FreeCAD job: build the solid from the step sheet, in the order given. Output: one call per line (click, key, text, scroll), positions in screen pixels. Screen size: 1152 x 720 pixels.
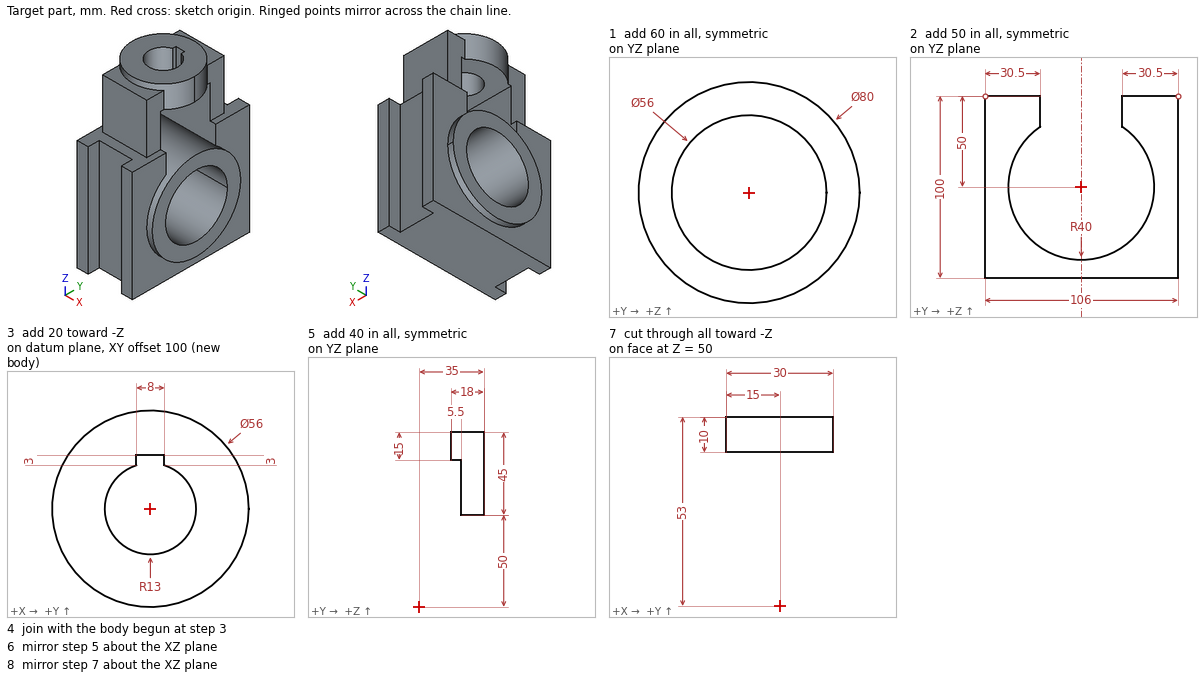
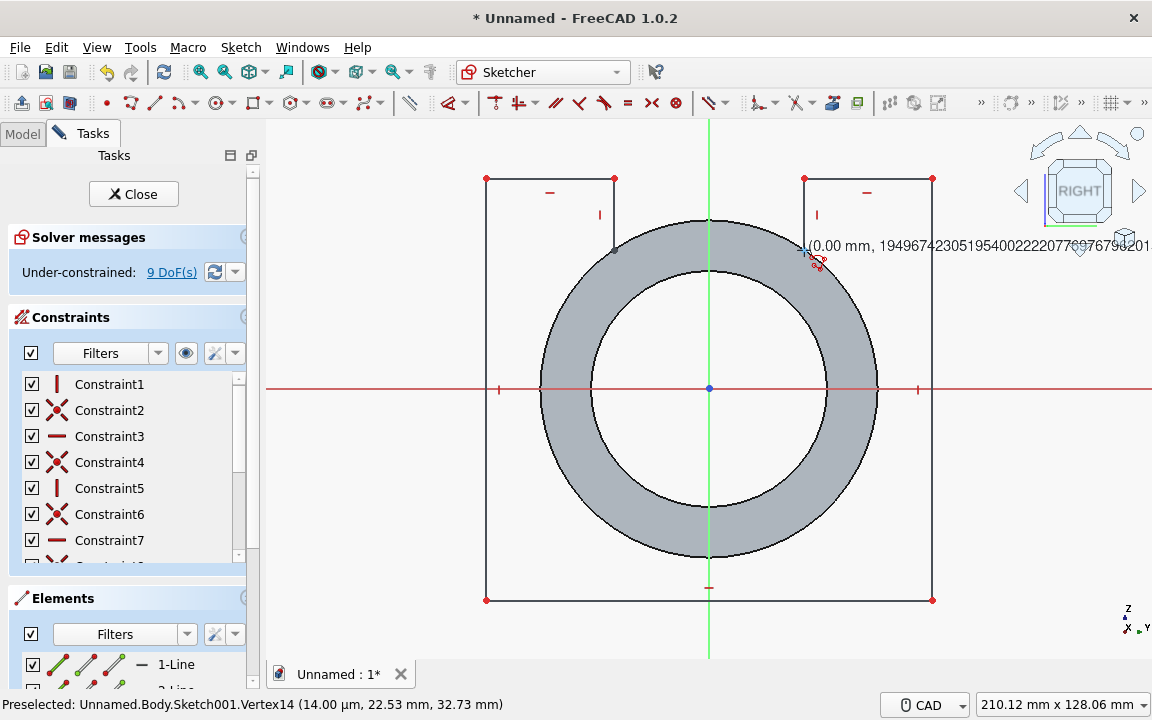
click(198, 104)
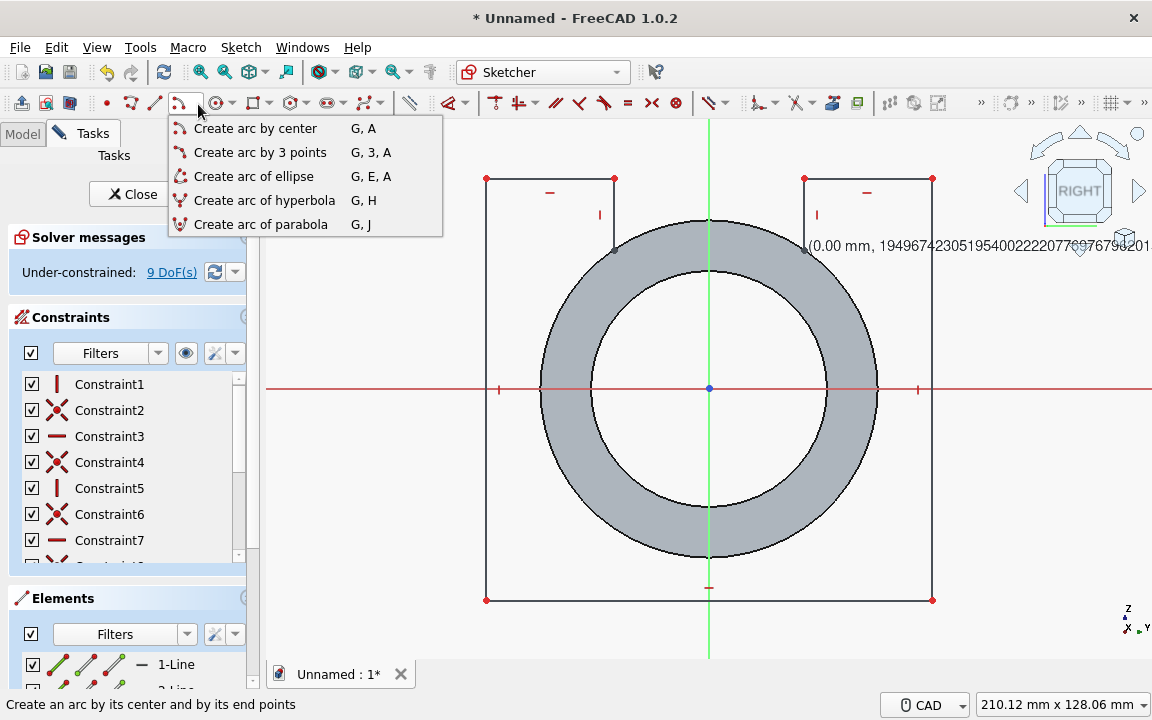
click(306, 152)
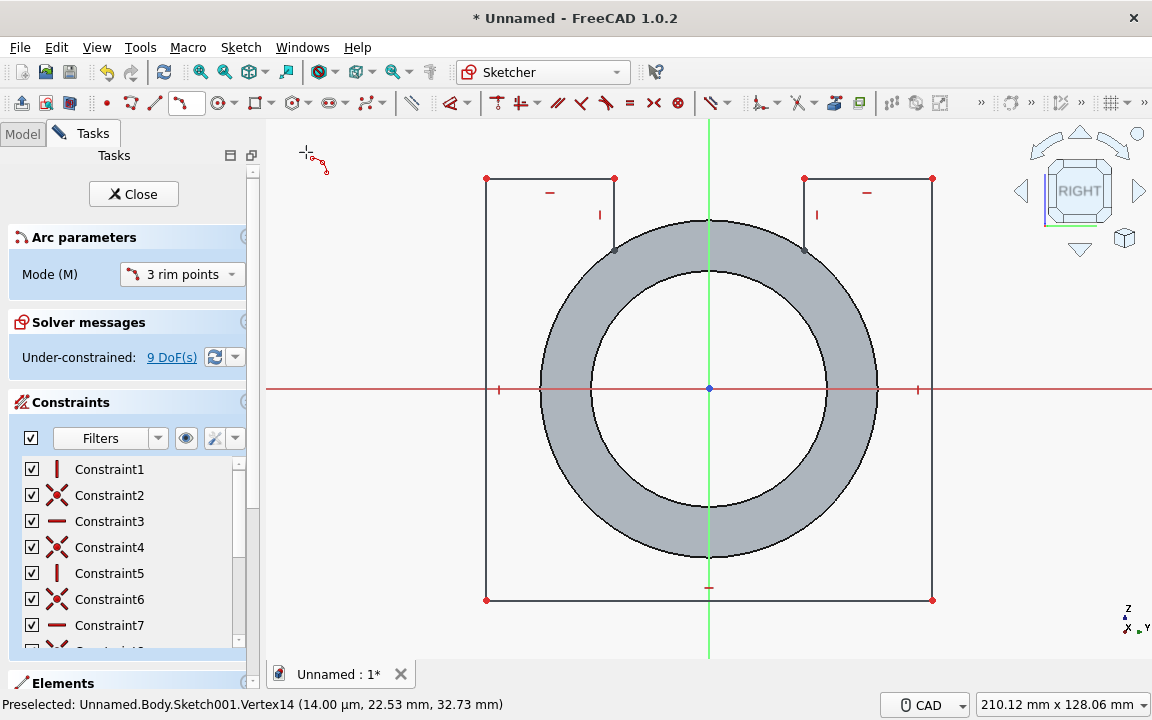
click(804, 251)
click(614, 251)
click(627, 536)
key(Escape)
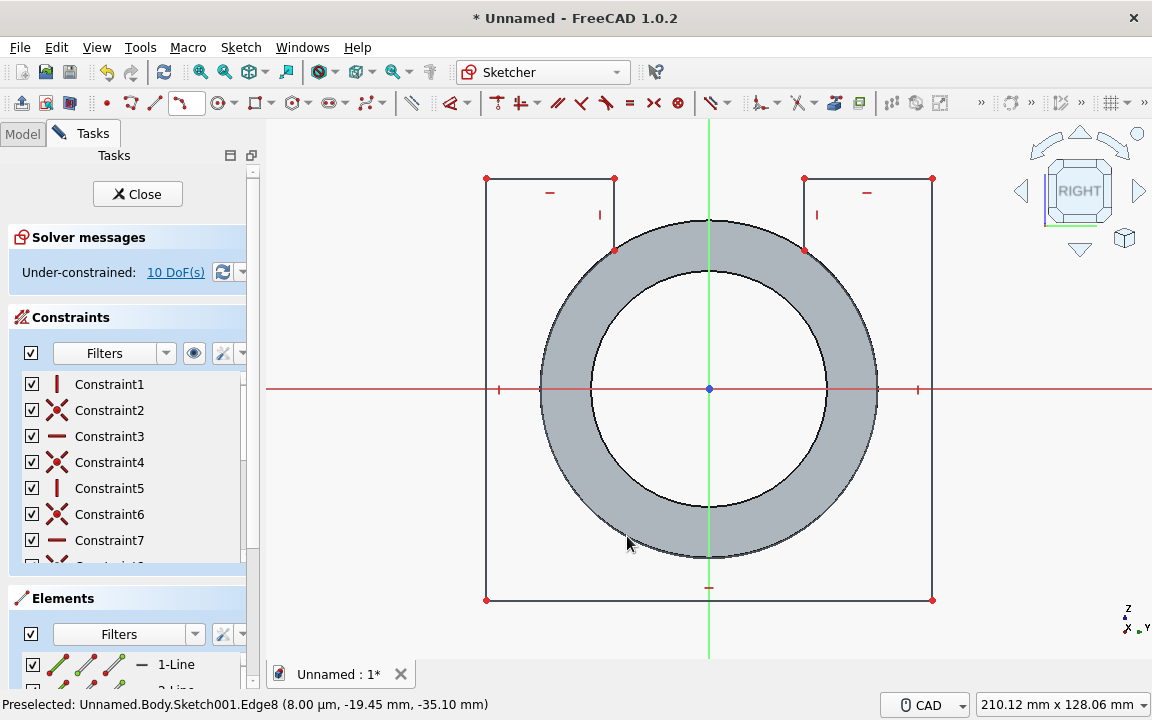
drag(699, 379, 719, 400)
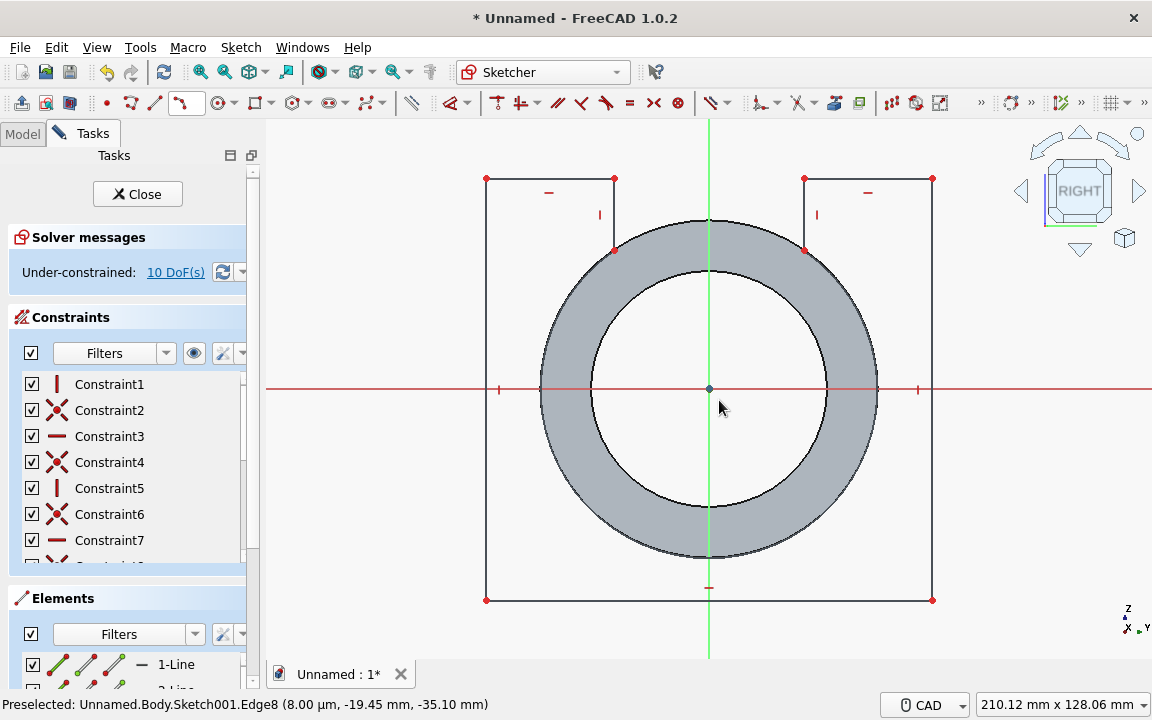
click(498, 104)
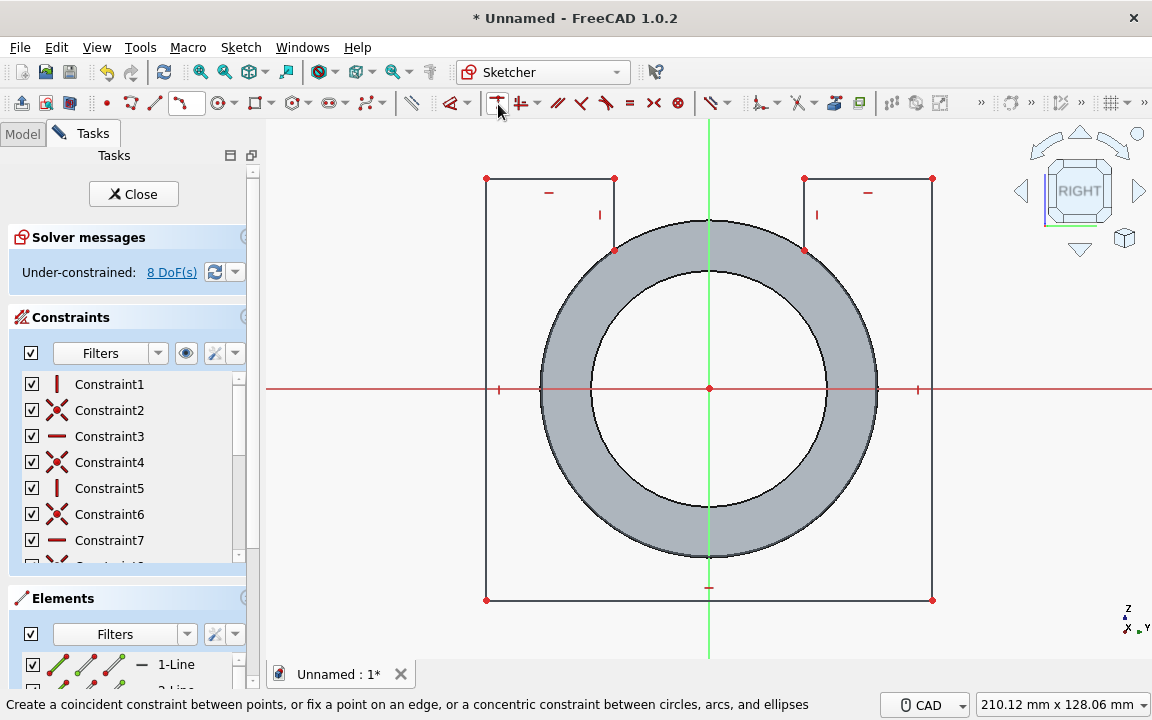
click(486, 179)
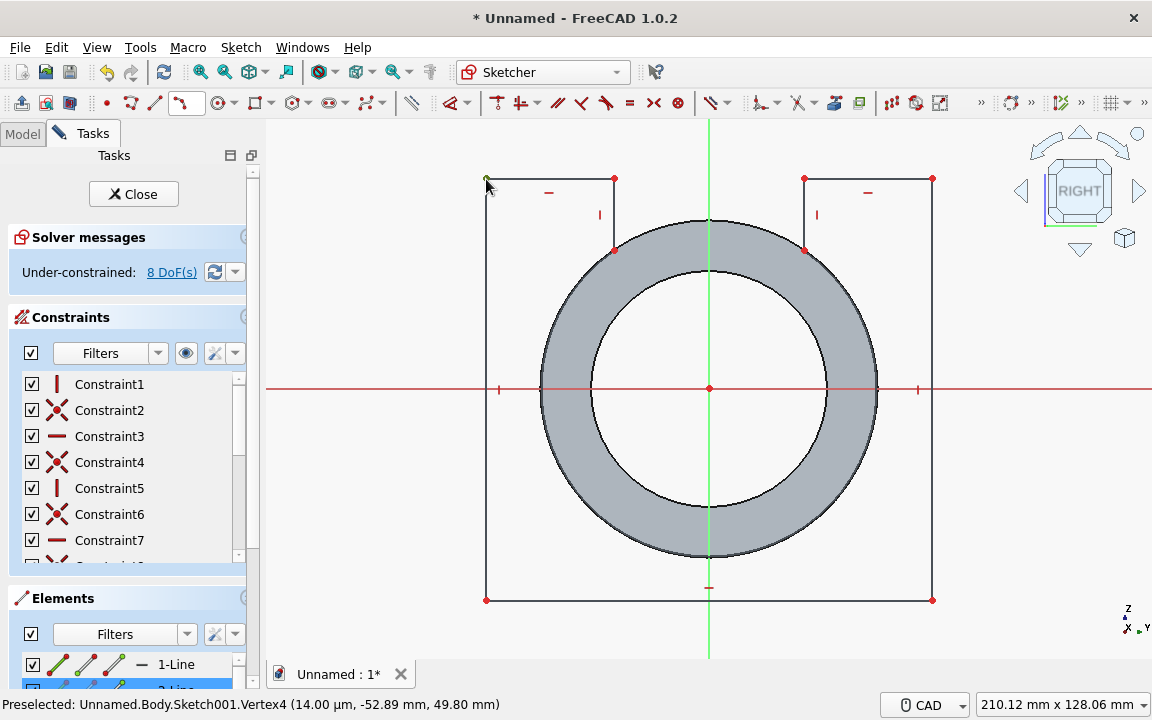
click(932, 179)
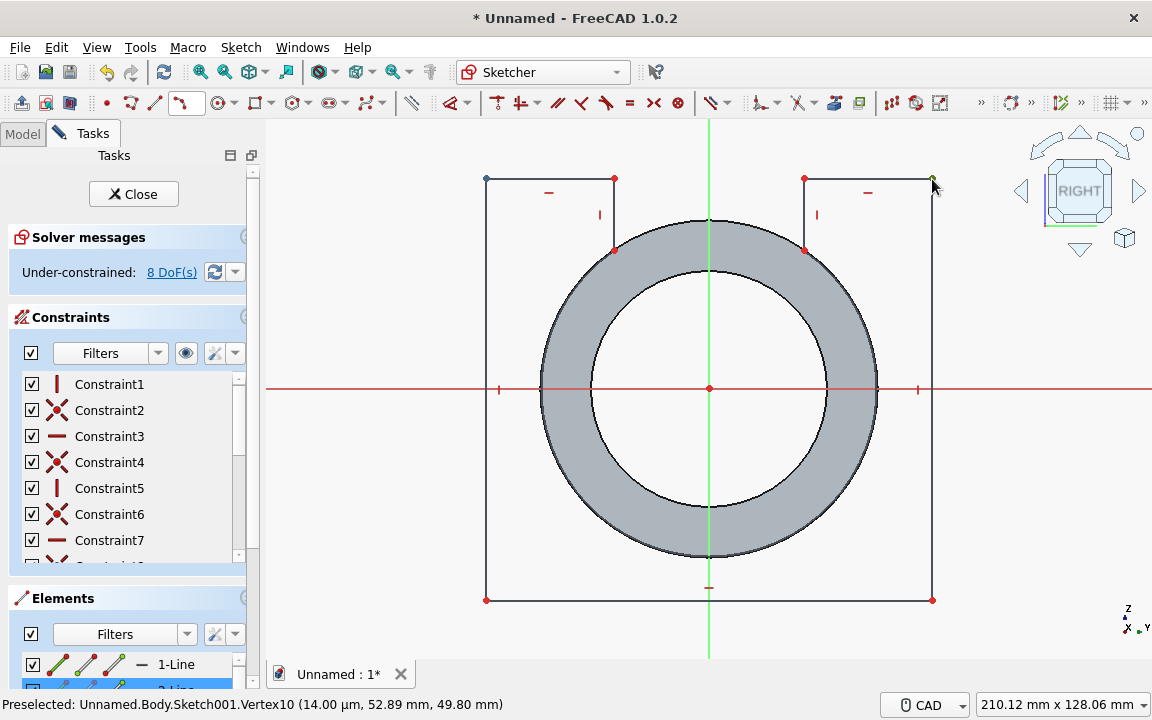
click(709, 493)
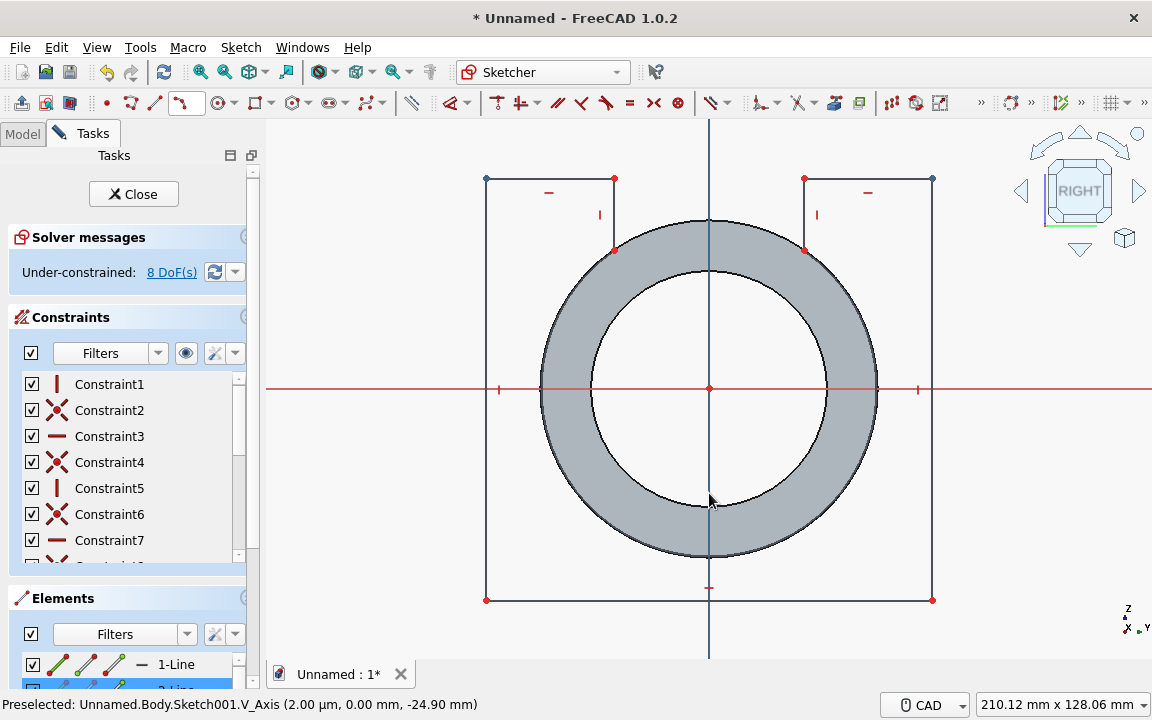
click(654, 104)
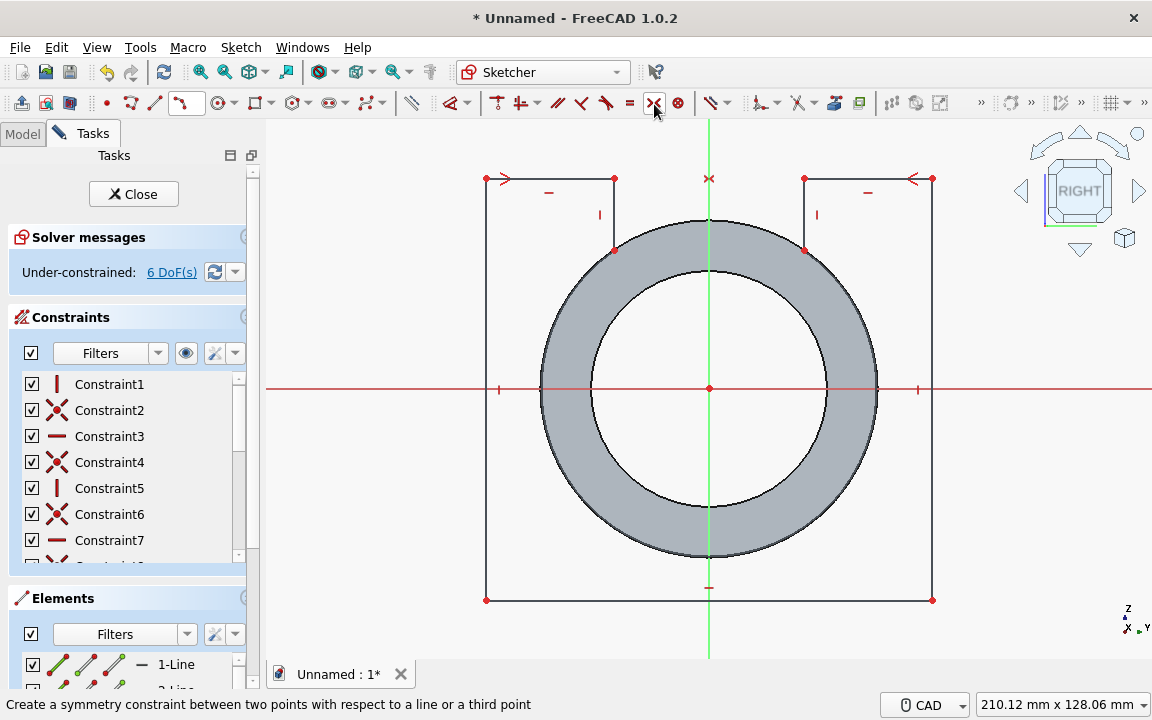
click(450, 104)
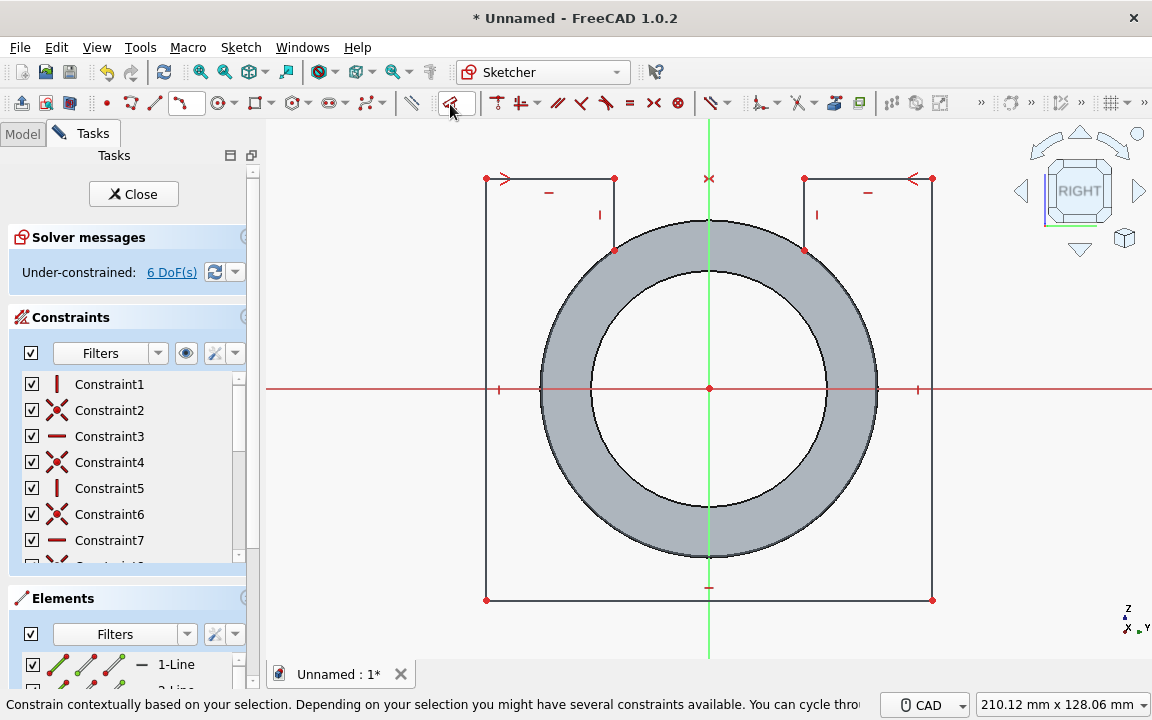
click(567, 477)
click(540, 494)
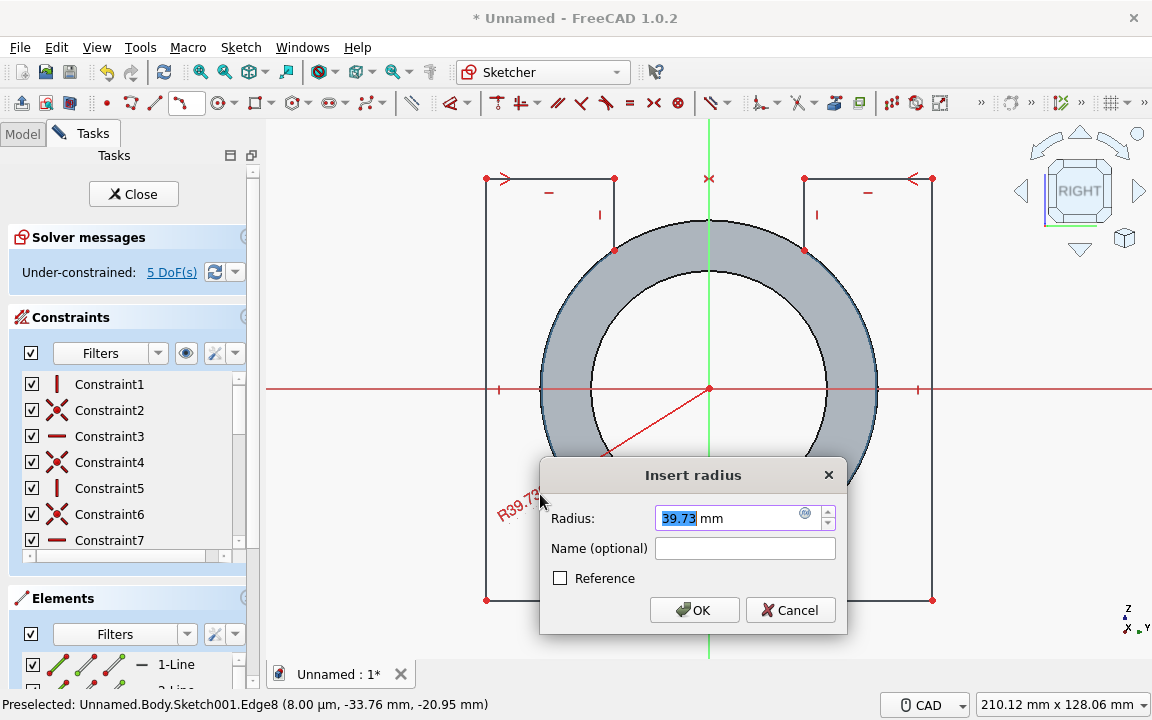
text(40)
key(Return)